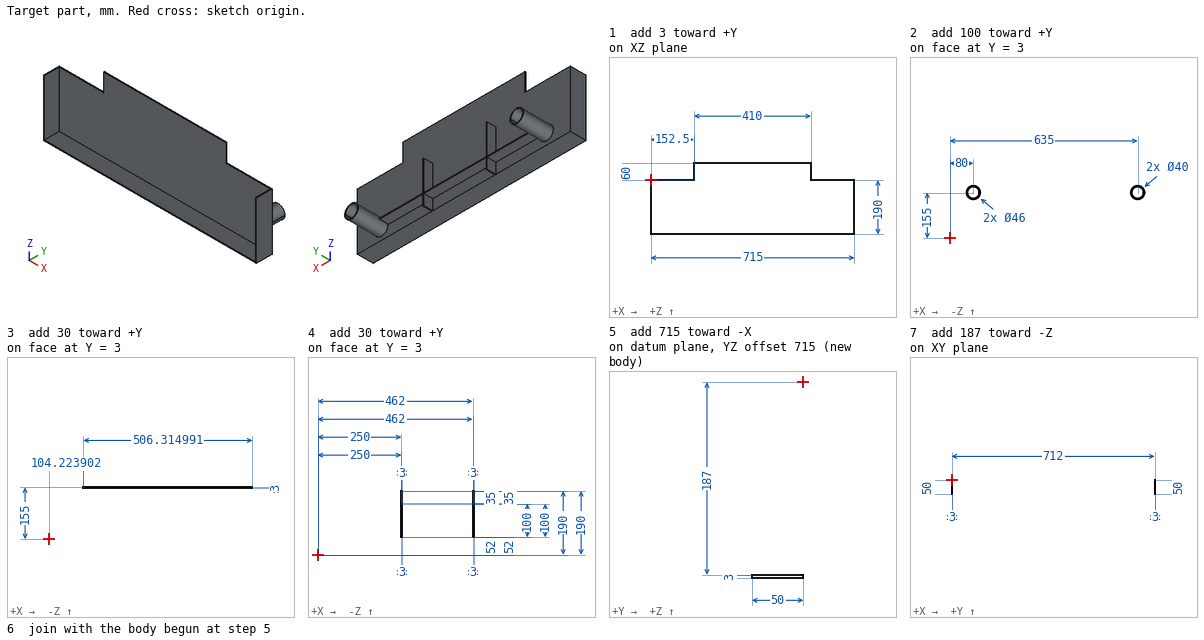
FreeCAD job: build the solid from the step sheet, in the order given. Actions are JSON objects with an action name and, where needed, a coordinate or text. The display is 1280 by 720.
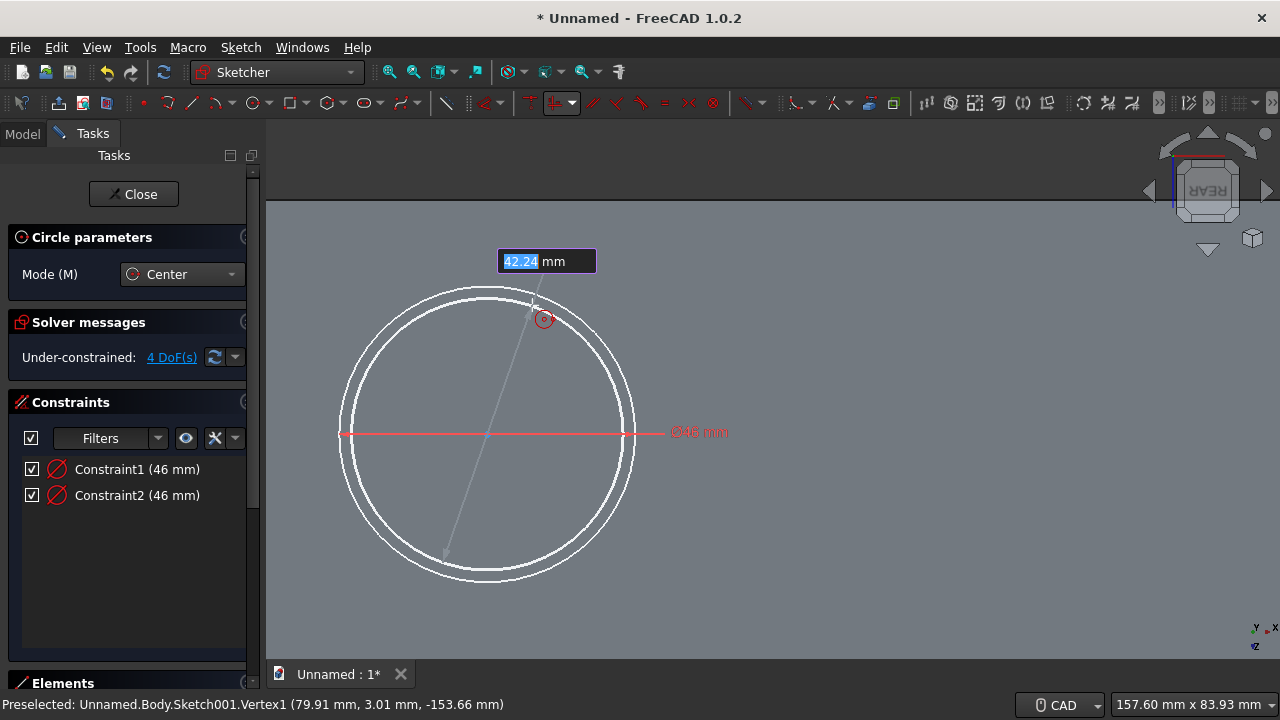
{"action": "type", "text": "40"}
{"action": "key", "text": "Return"}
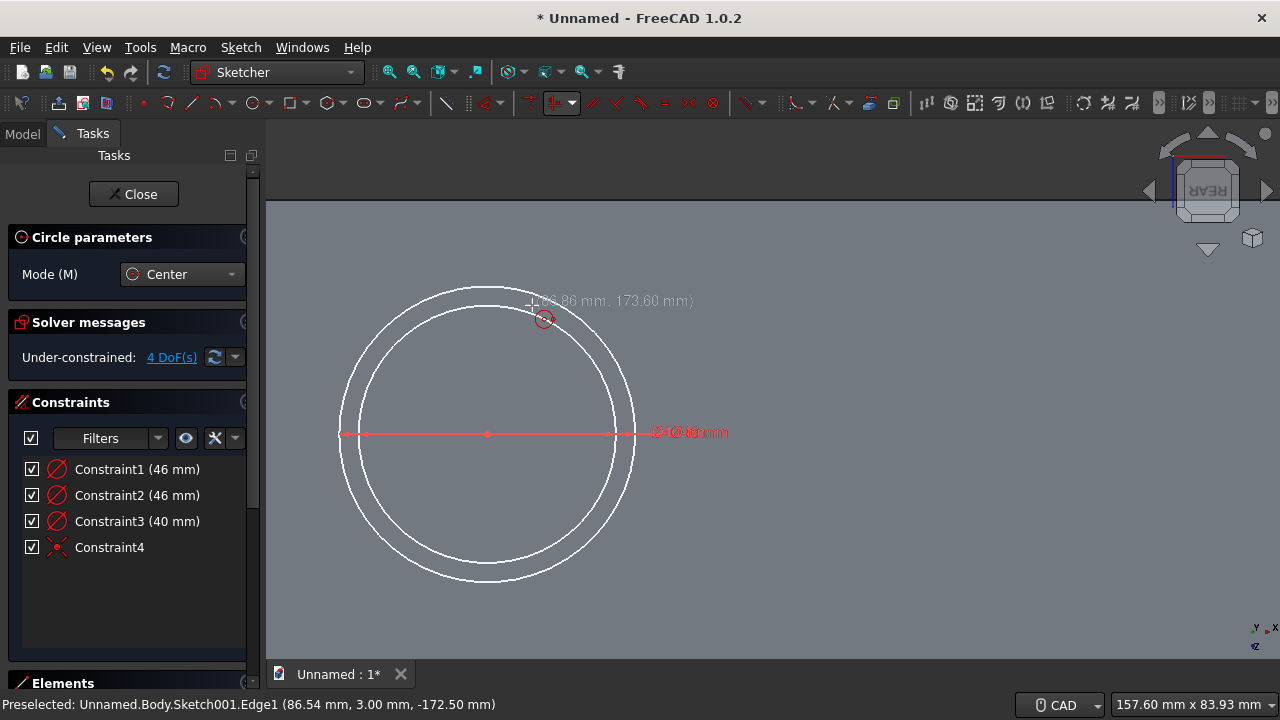
{"action": "scroll", "coordinate": [488, 317], "scroll_direction": "down", "scroll_amount": 10}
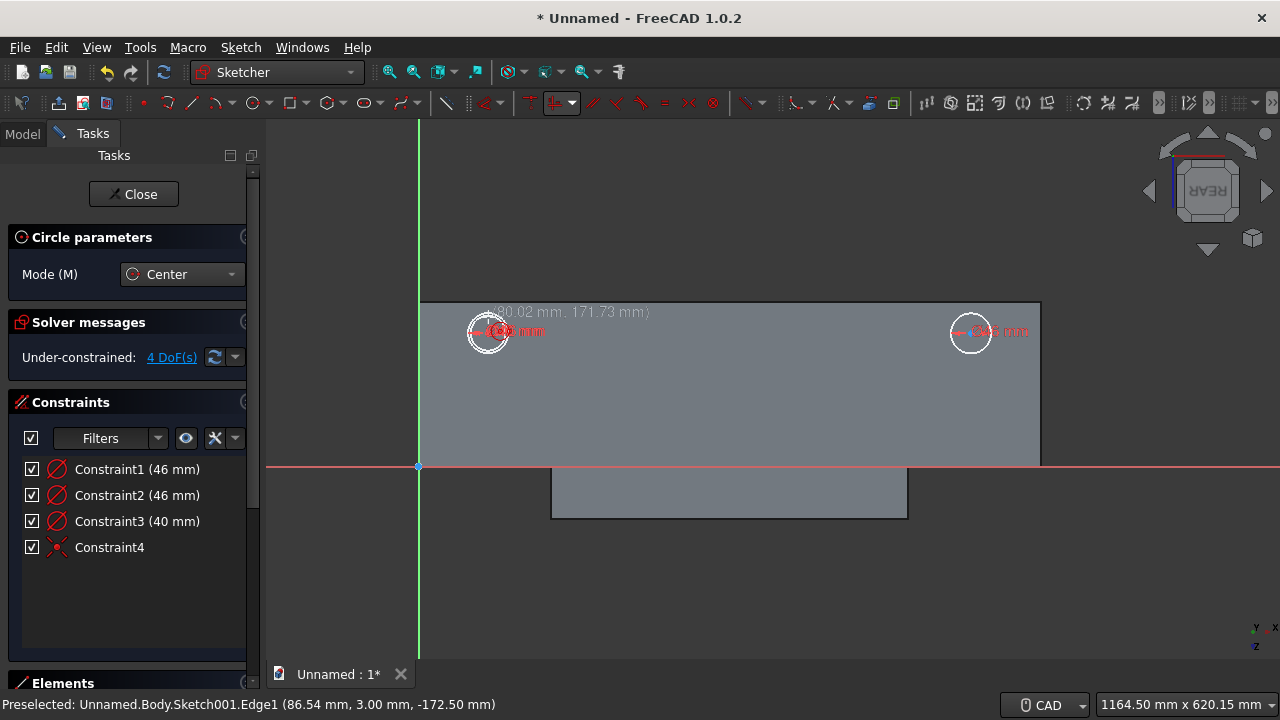
{"action": "scroll", "coordinate": [971, 332], "scroll_direction": "up", "scroll_amount": 2}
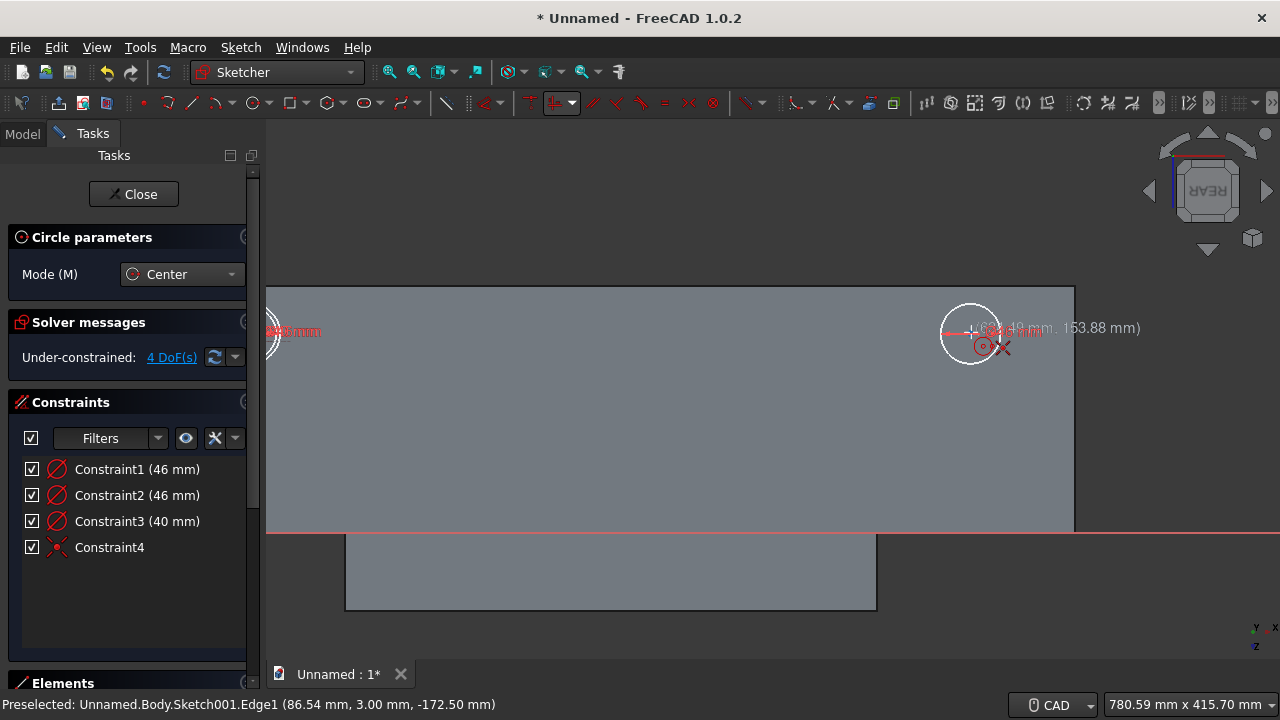
{"action": "left_click", "coordinate": [971, 334]}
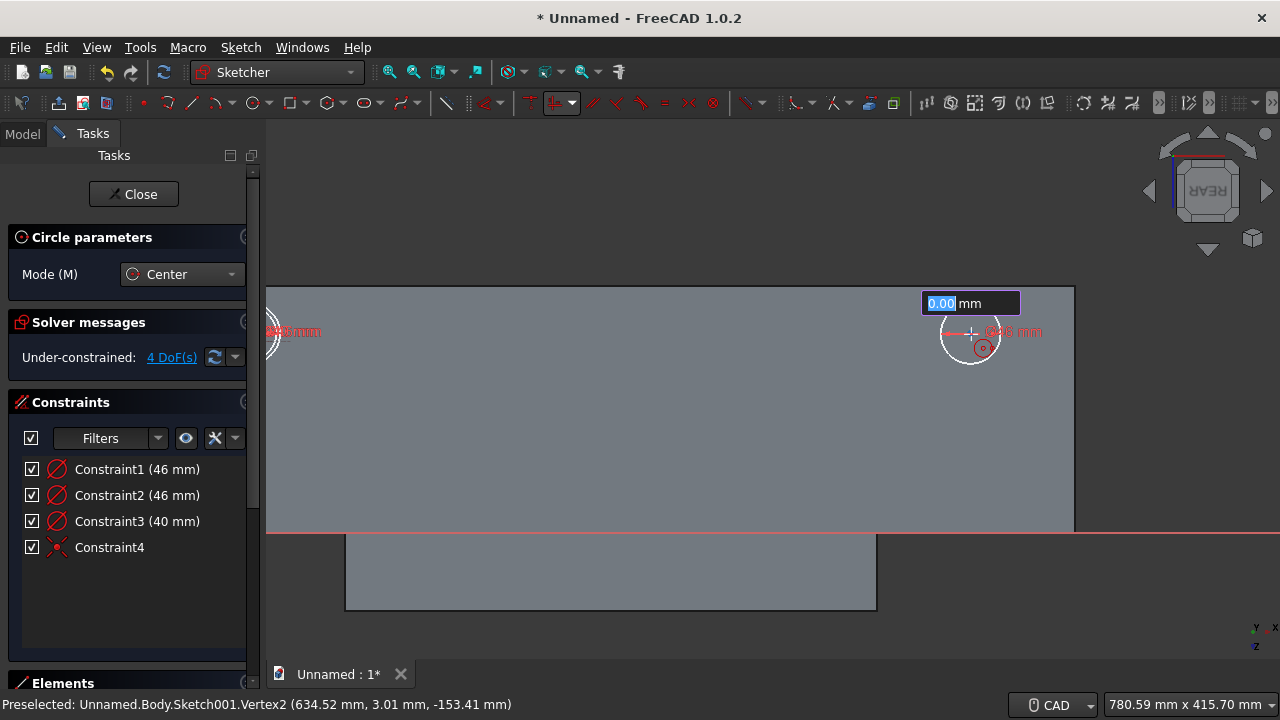
{"action": "scroll", "coordinate": [990, 313], "scroll_direction": "up", "scroll_amount": 8}
{"action": "mouse_move", "coordinate": [986, 314]}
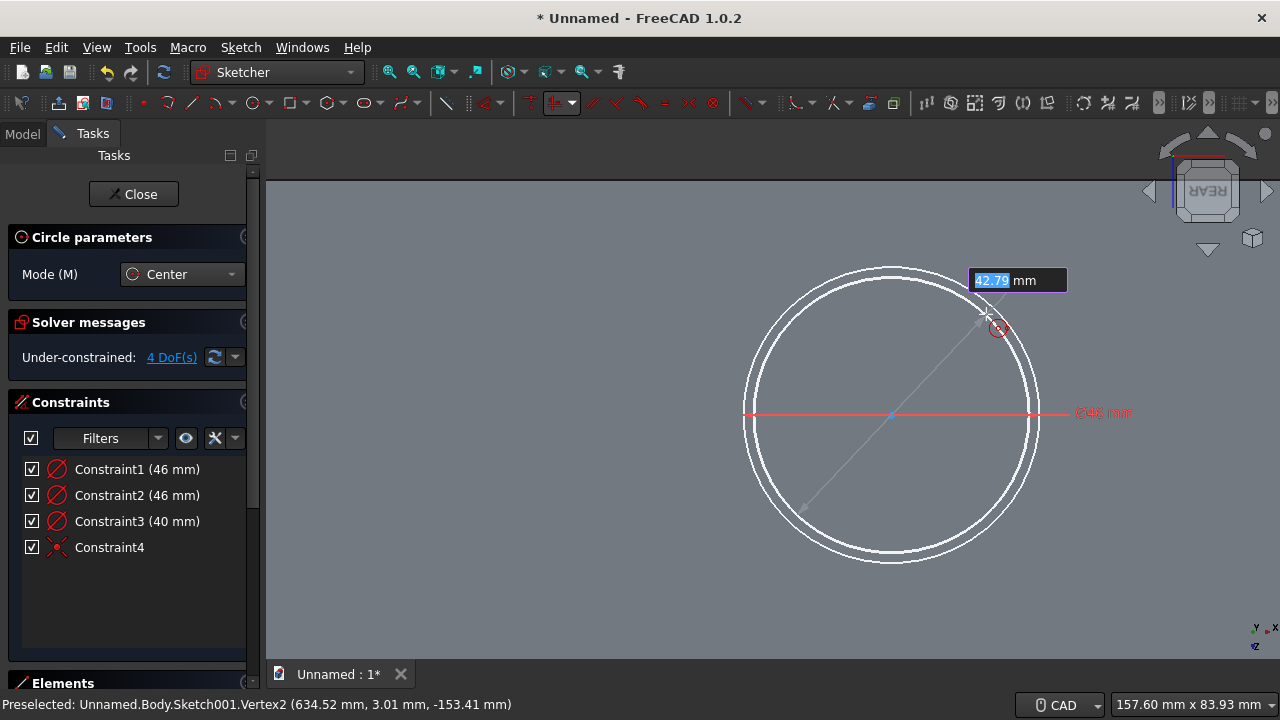
{"action": "type", "text": "40"}
{"action": "key", "text": "Return"}
{"action": "key", "text": "Escape"}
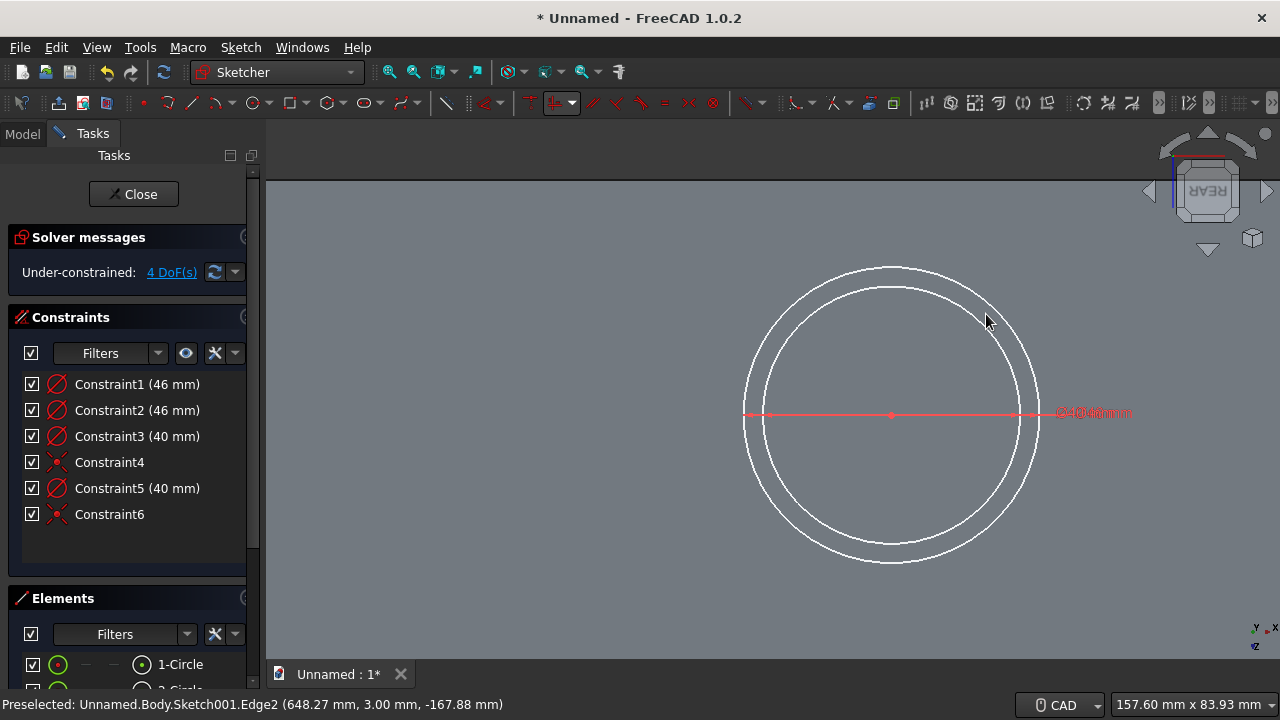
{"action": "scroll", "coordinate": [983, 320], "scroll_direction": "down", "scroll_amount": 10}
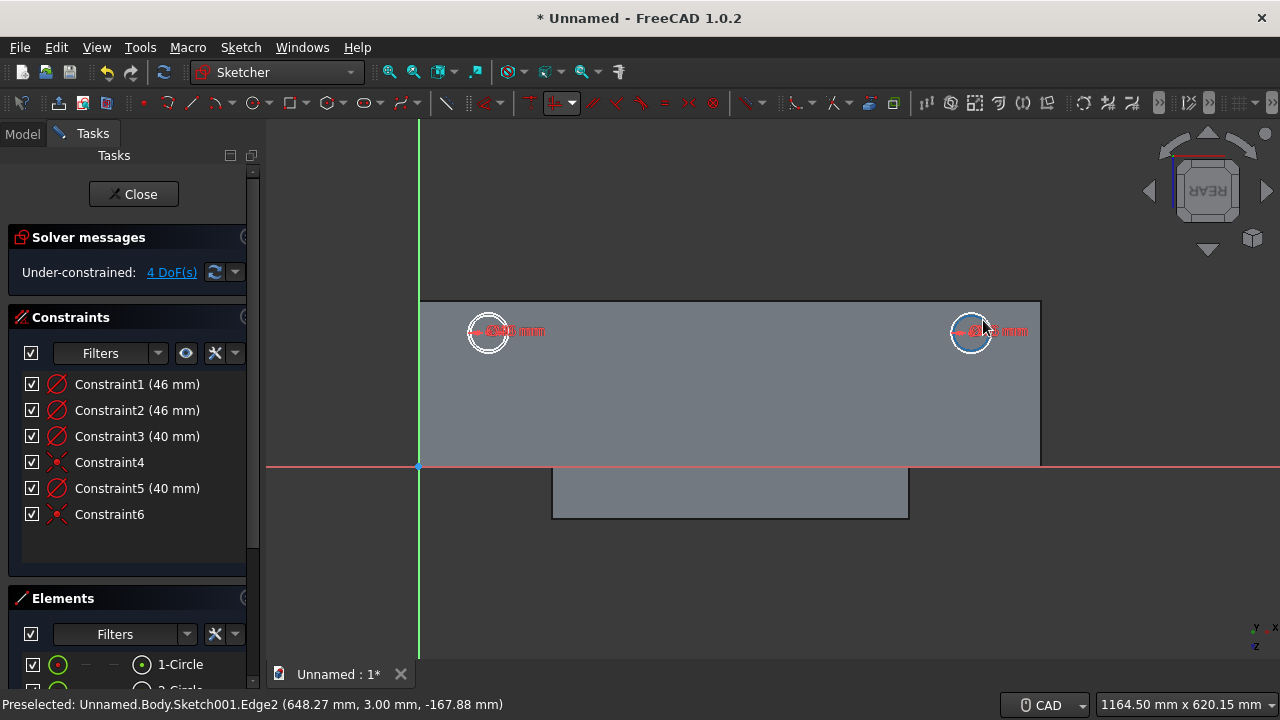
{"action": "left_click", "coordinate": [488, 333]}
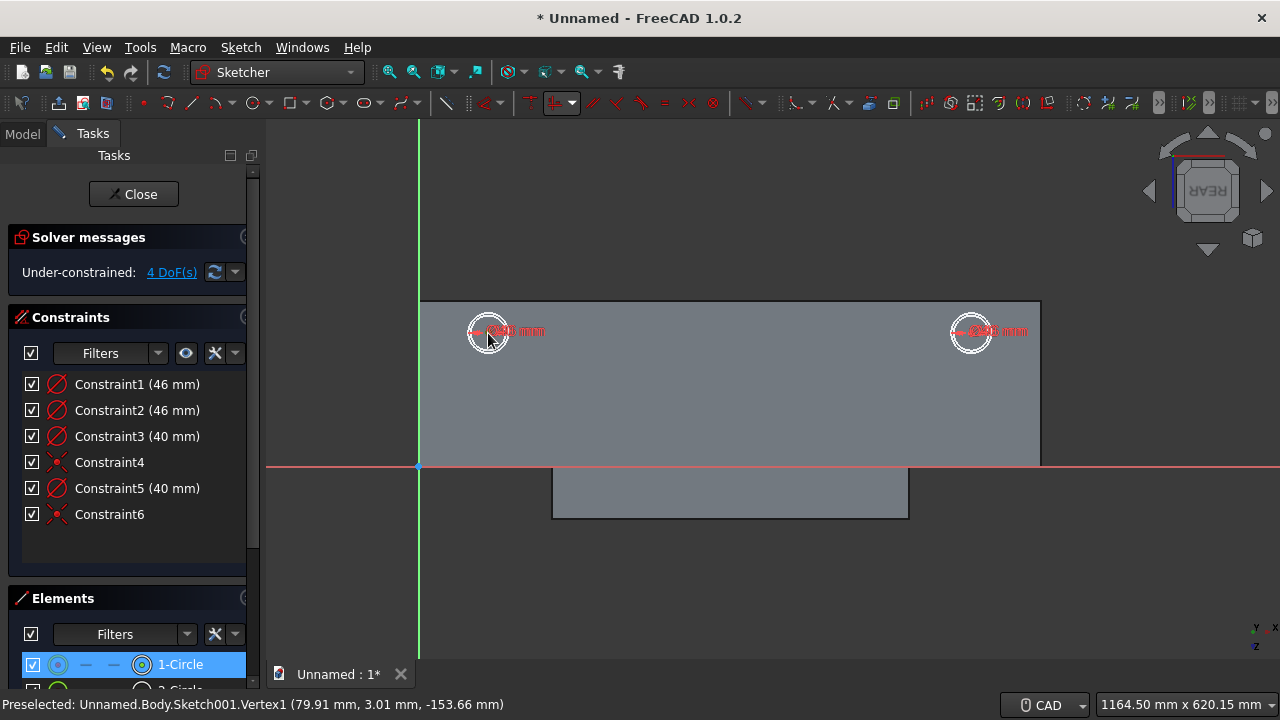
{"action": "left_click", "coordinate": [971, 333]}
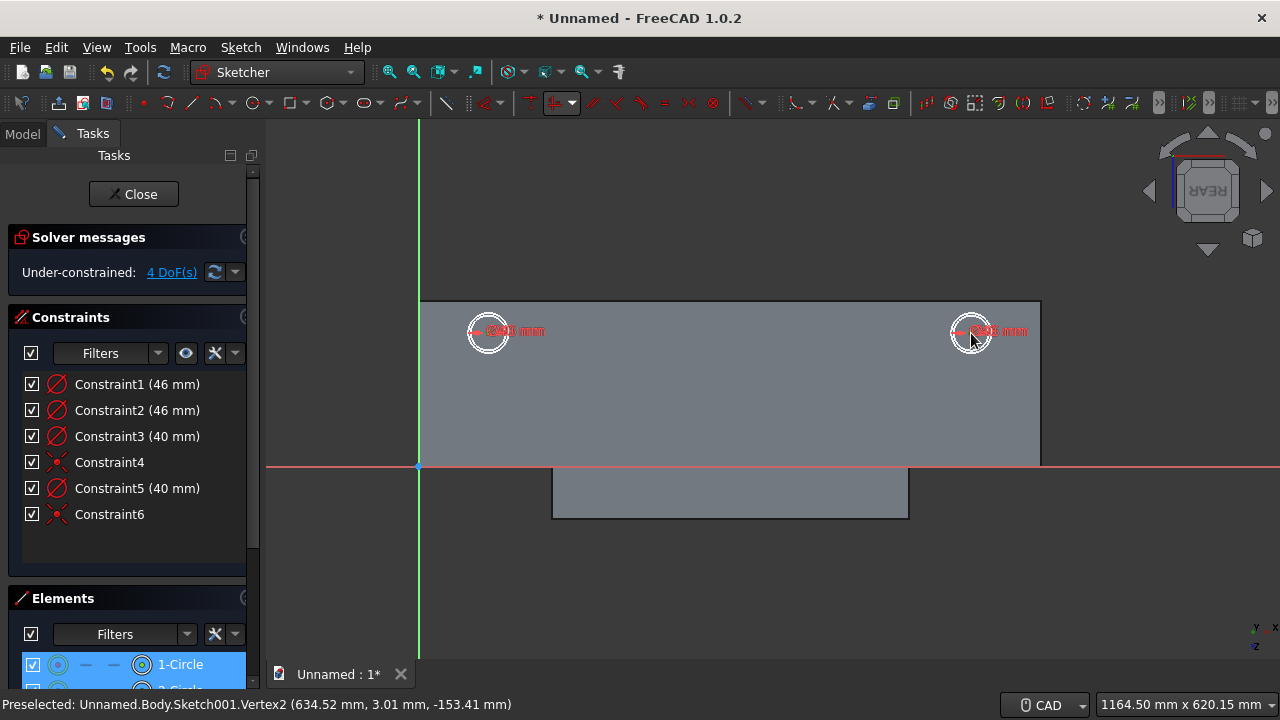
{"action": "left_click", "coordinate": [574, 104]}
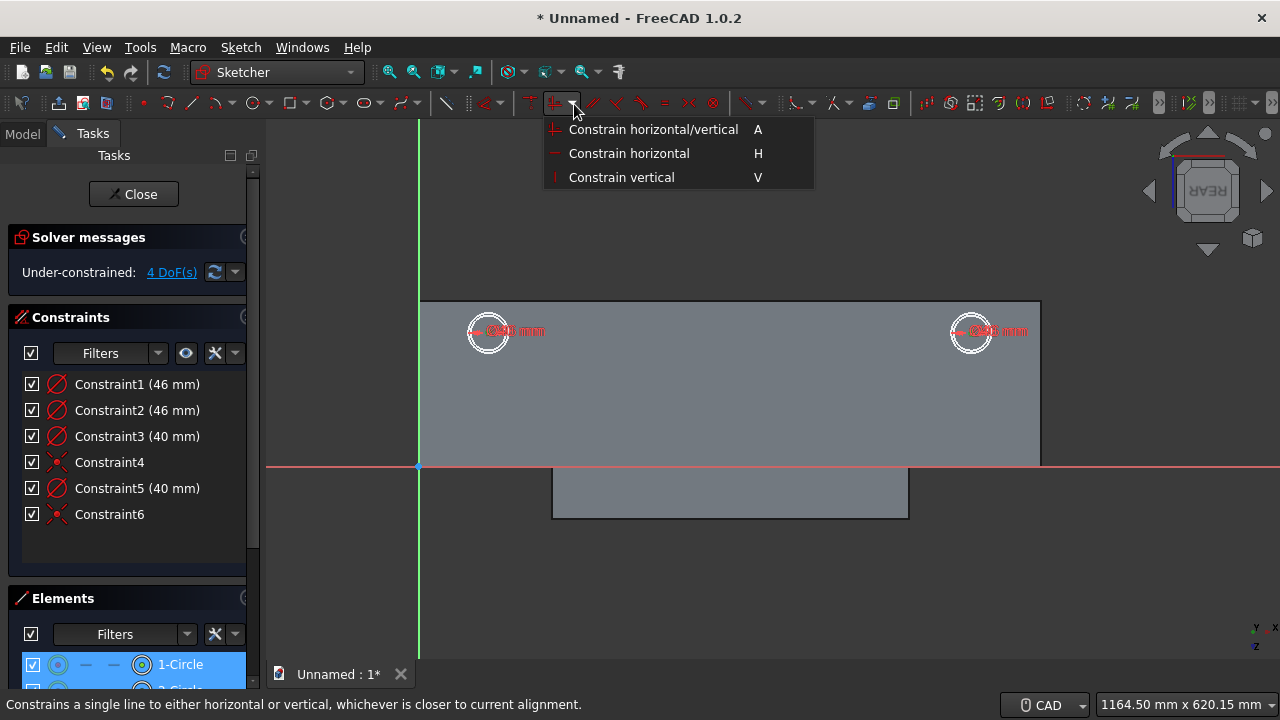
{"action": "left_click", "coordinate": [679, 153]}